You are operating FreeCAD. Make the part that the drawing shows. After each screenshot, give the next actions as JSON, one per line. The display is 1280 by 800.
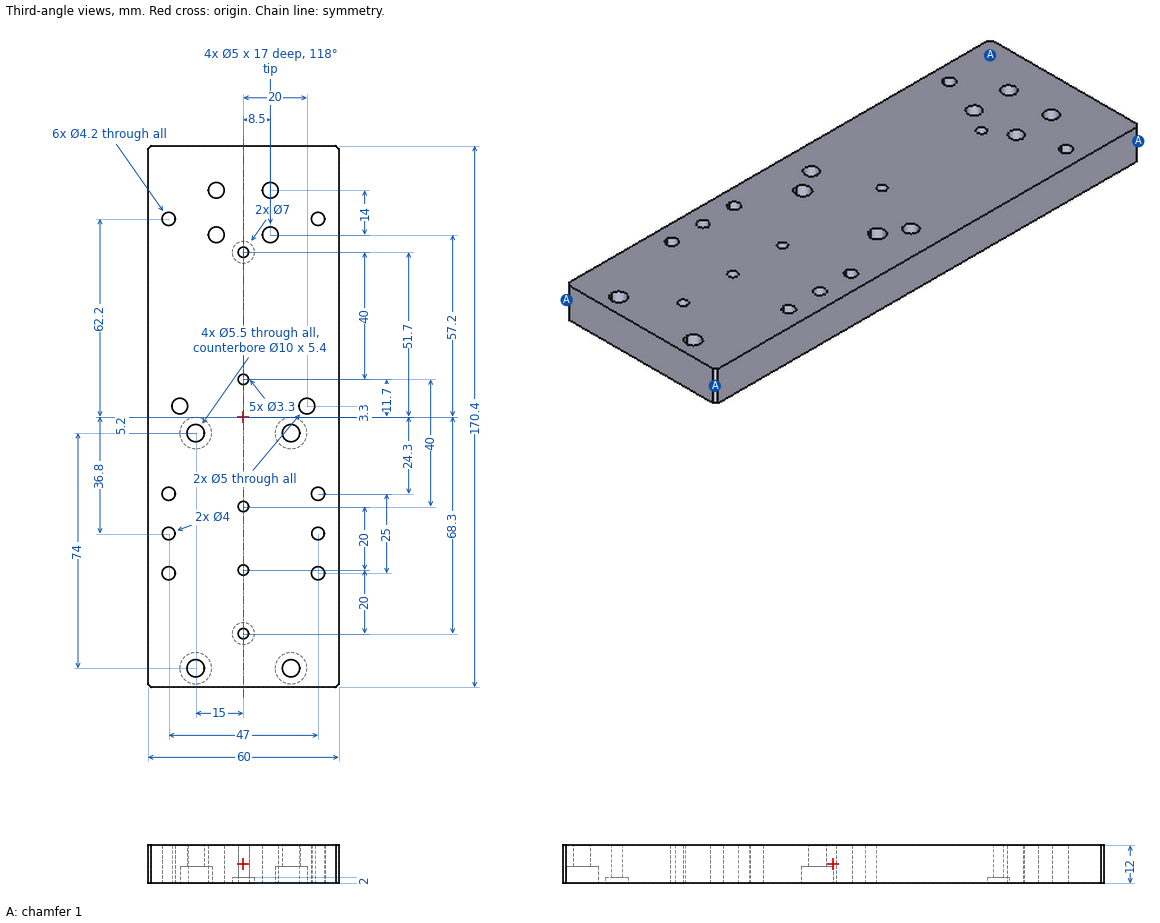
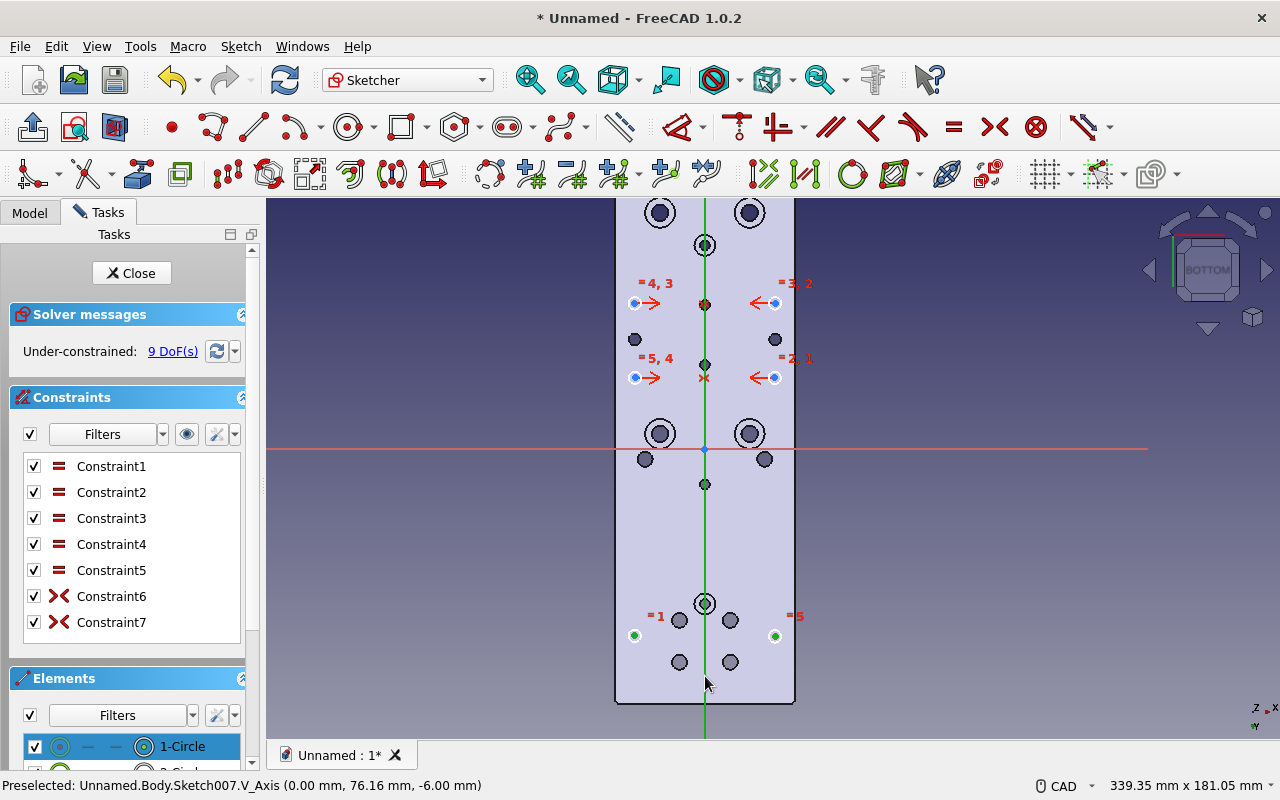
{"action": "left_click", "coordinate": [995, 128]}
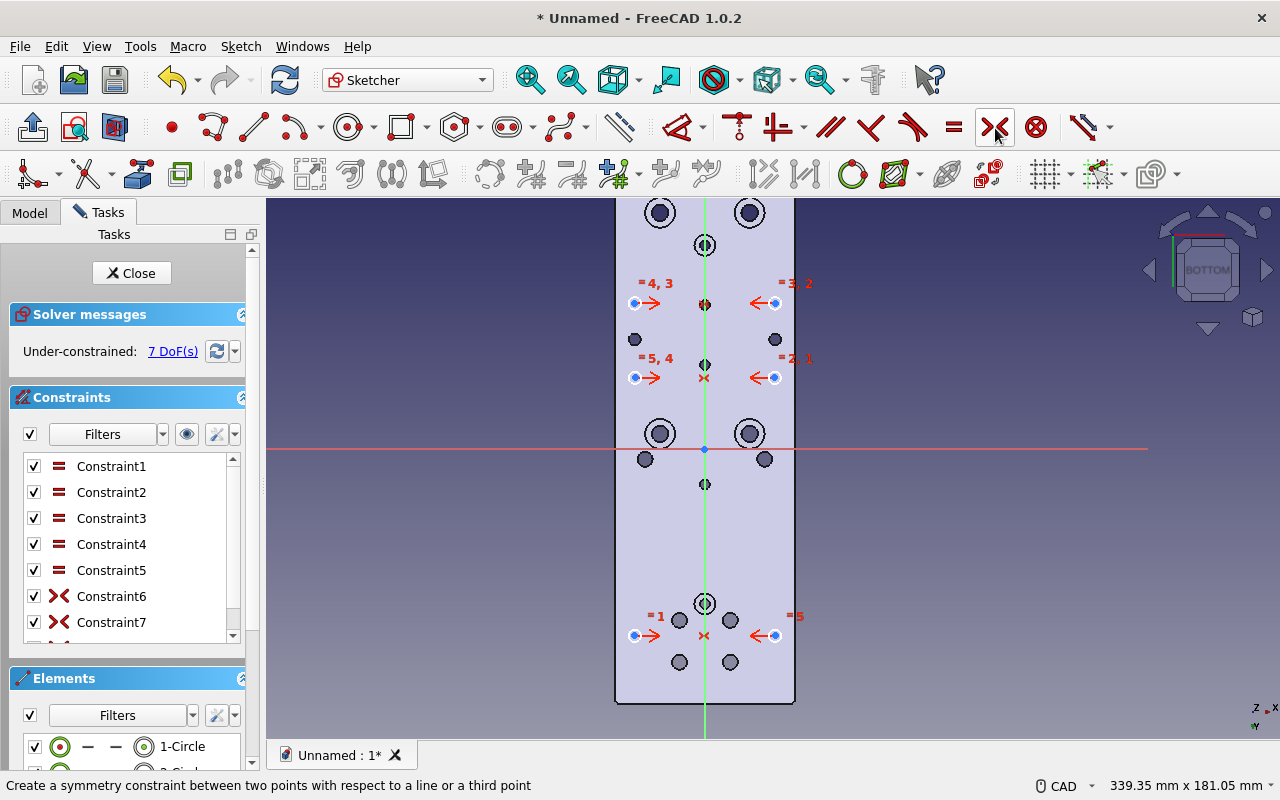
{"action": "left_click", "coordinate": [676, 128]}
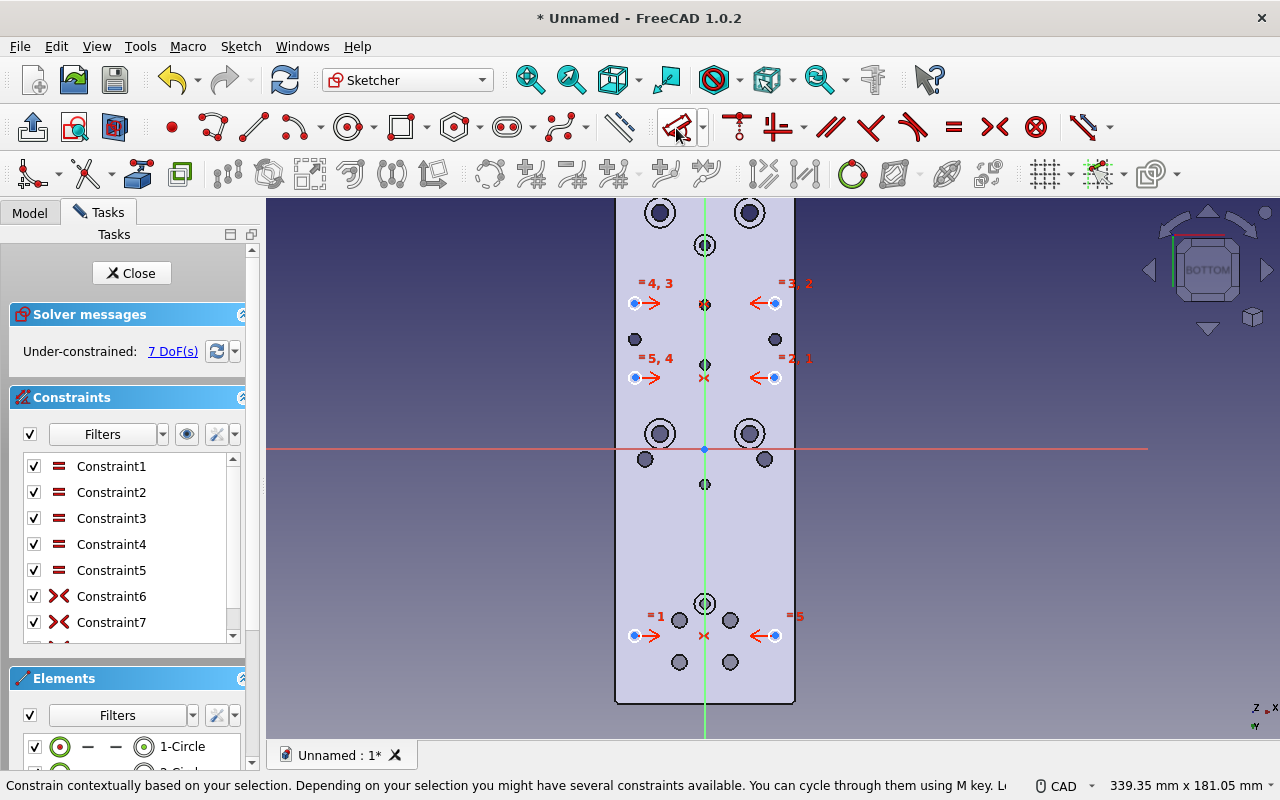
{"action": "scroll", "coordinate": [635, 642], "scroll_direction": "up", "scroll_amount": 6}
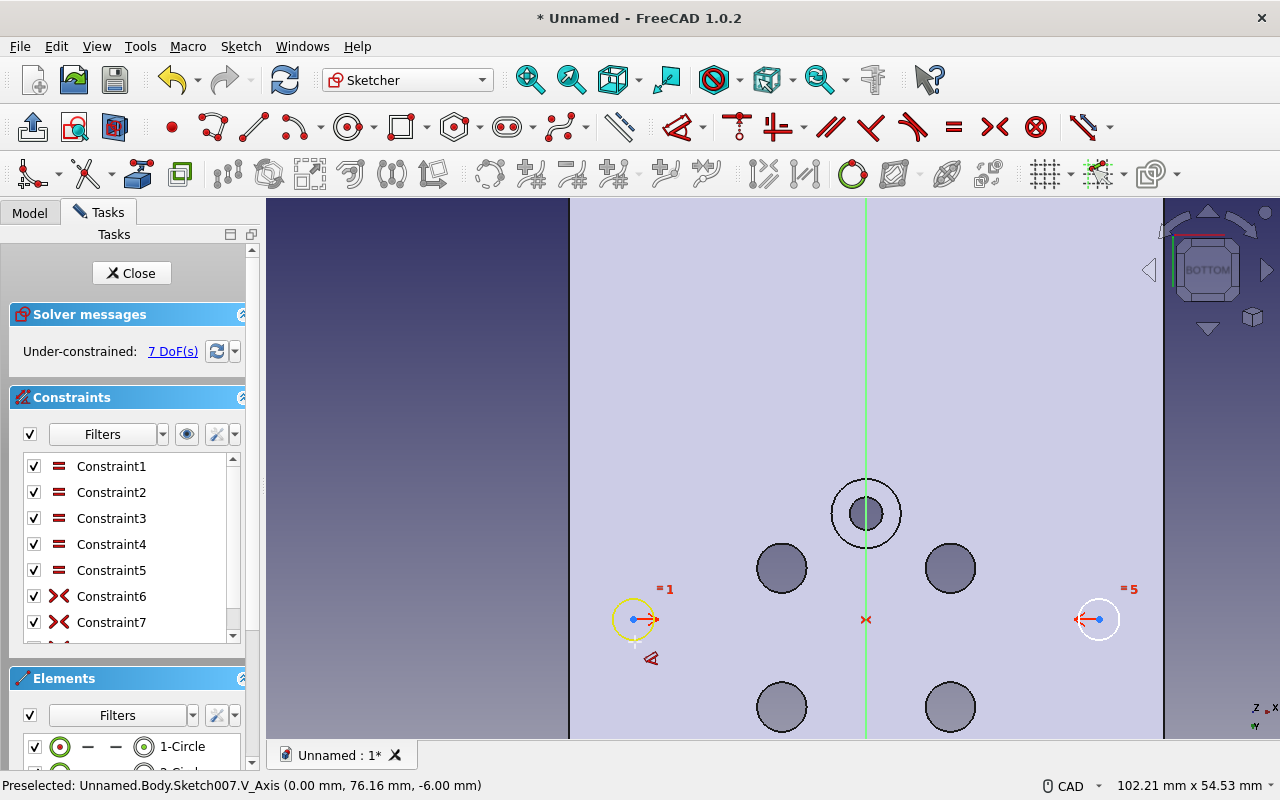
{"action": "left_click", "coordinate": [633, 640]}
{"action": "left_click", "coordinate": [632, 672]}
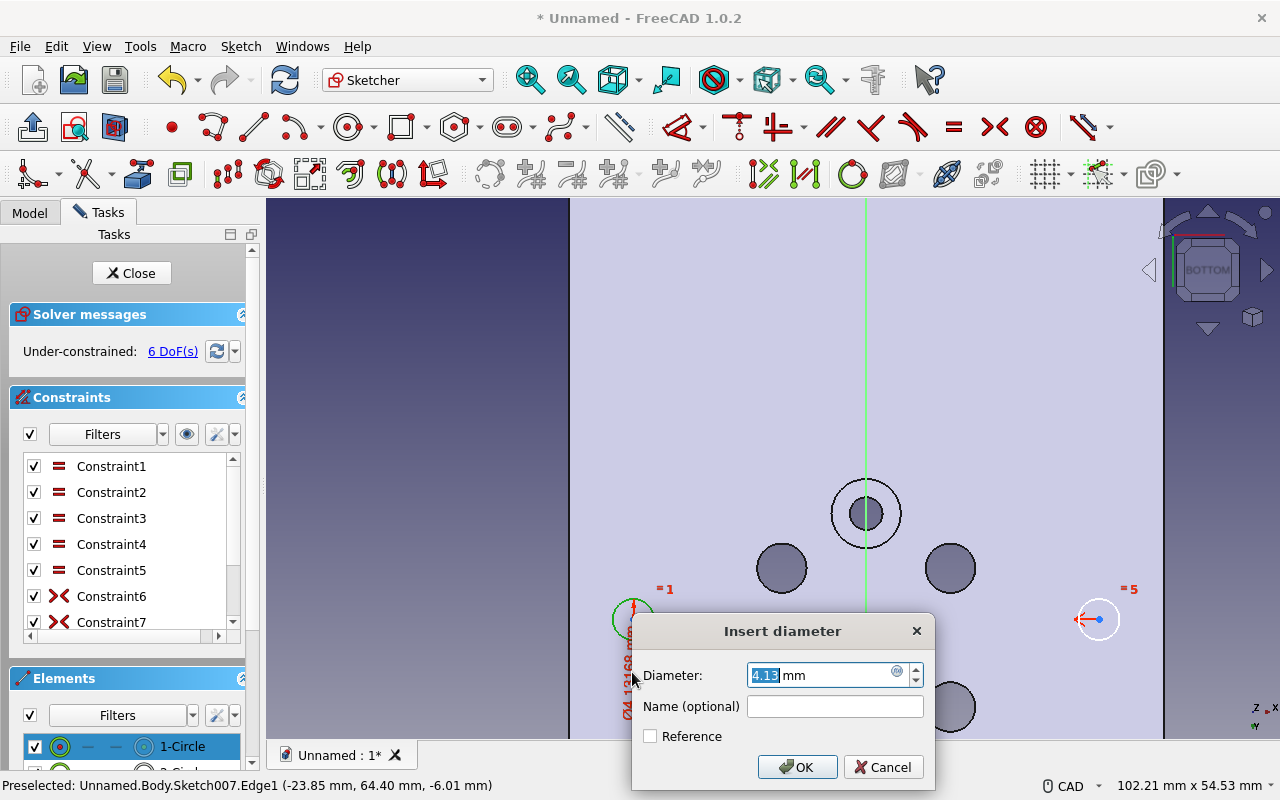
{"action": "type", "text": "4.2"}
{"action": "key", "text": "Return"}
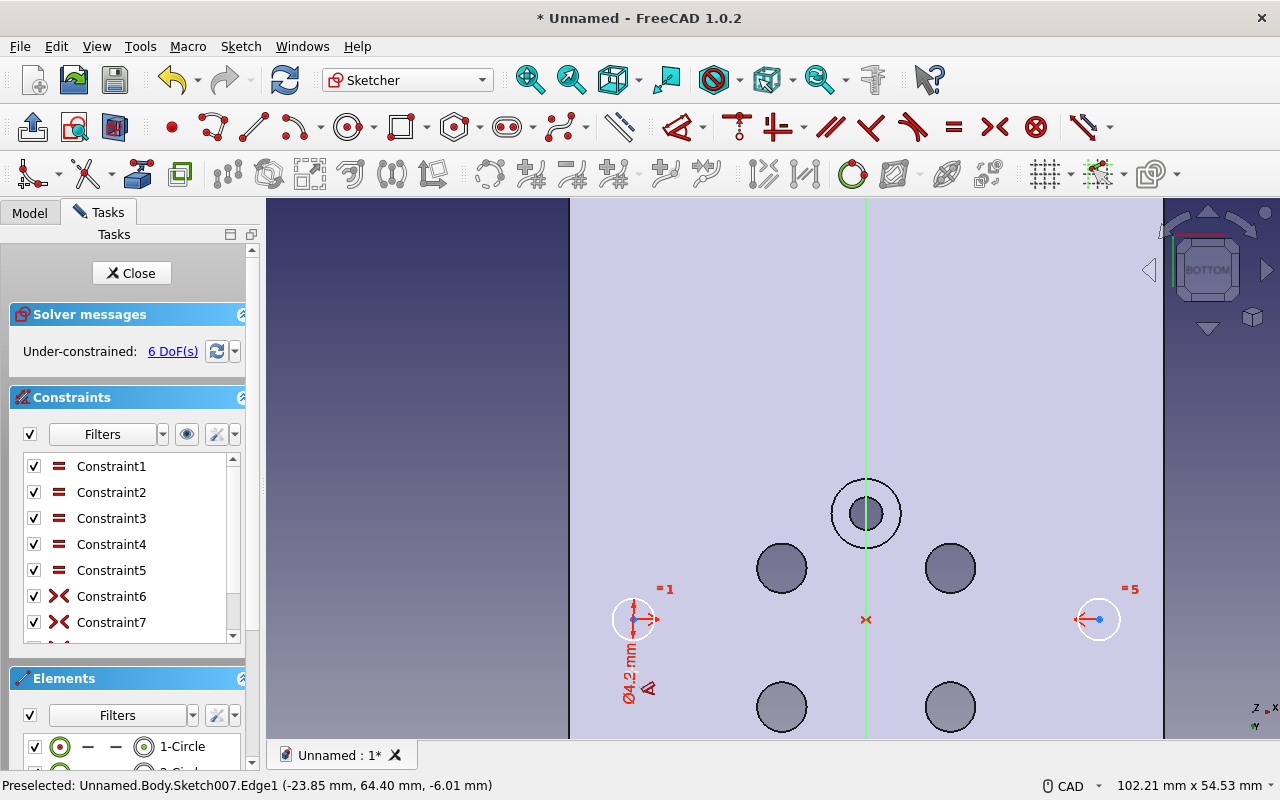
{"action": "left_click", "coordinate": [633, 619]}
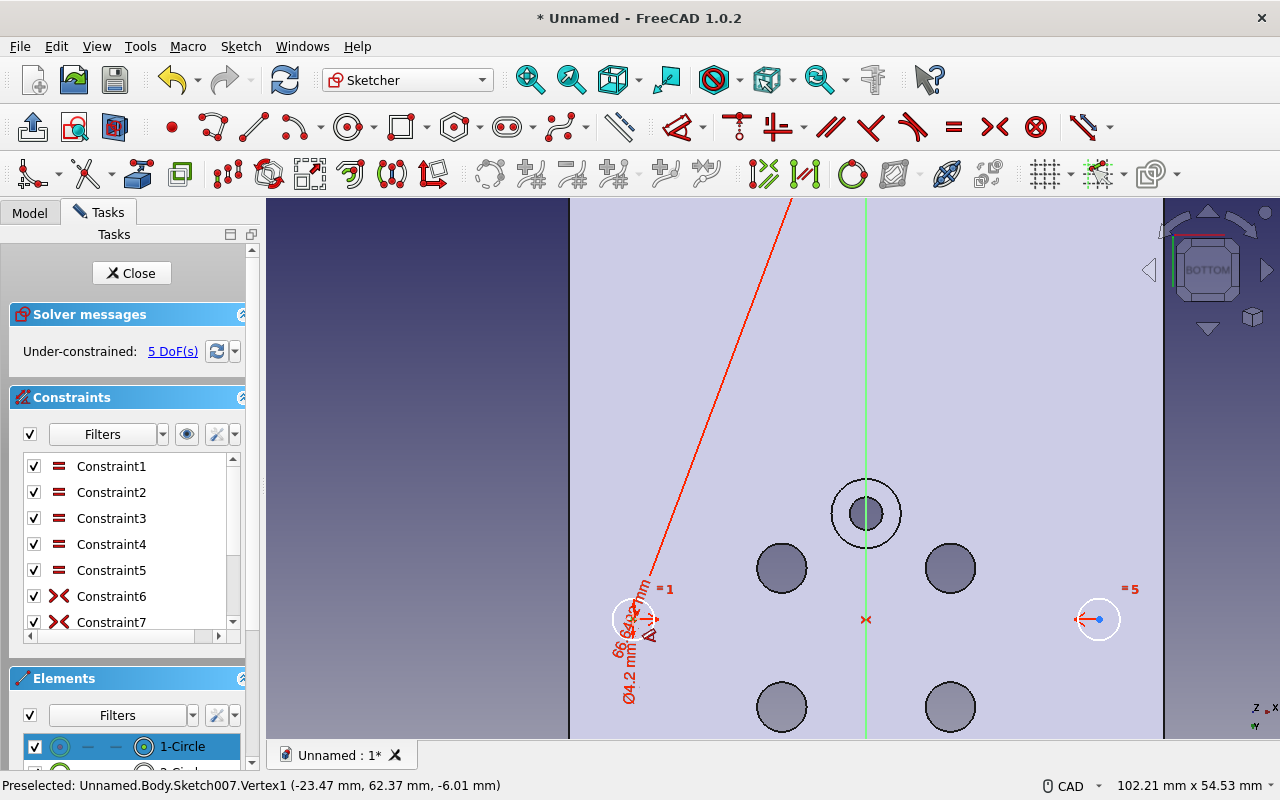
{"action": "scroll", "coordinate": [635, 643], "scroll_direction": "down", "scroll_amount": 6}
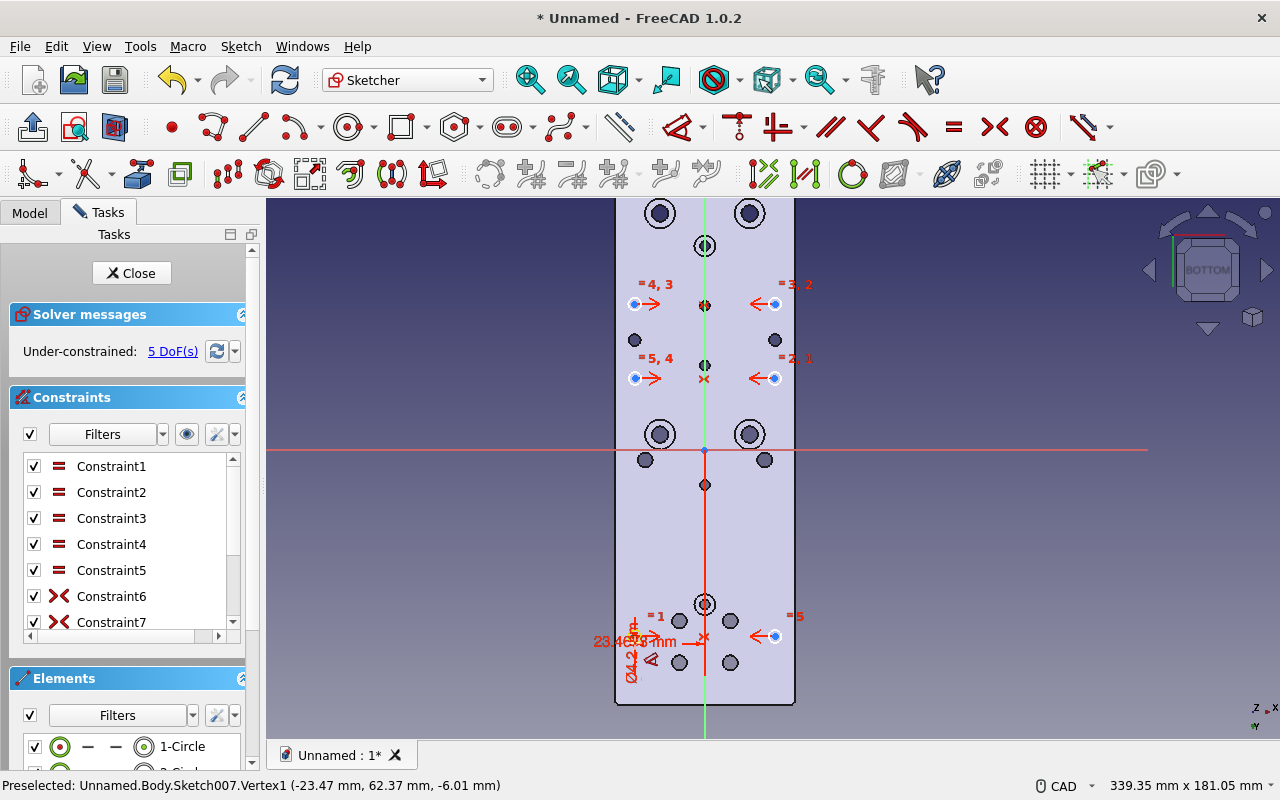
{"action": "left_click", "coordinate": [775, 378]}
{"action": "left_click", "coordinate": [737, 670]}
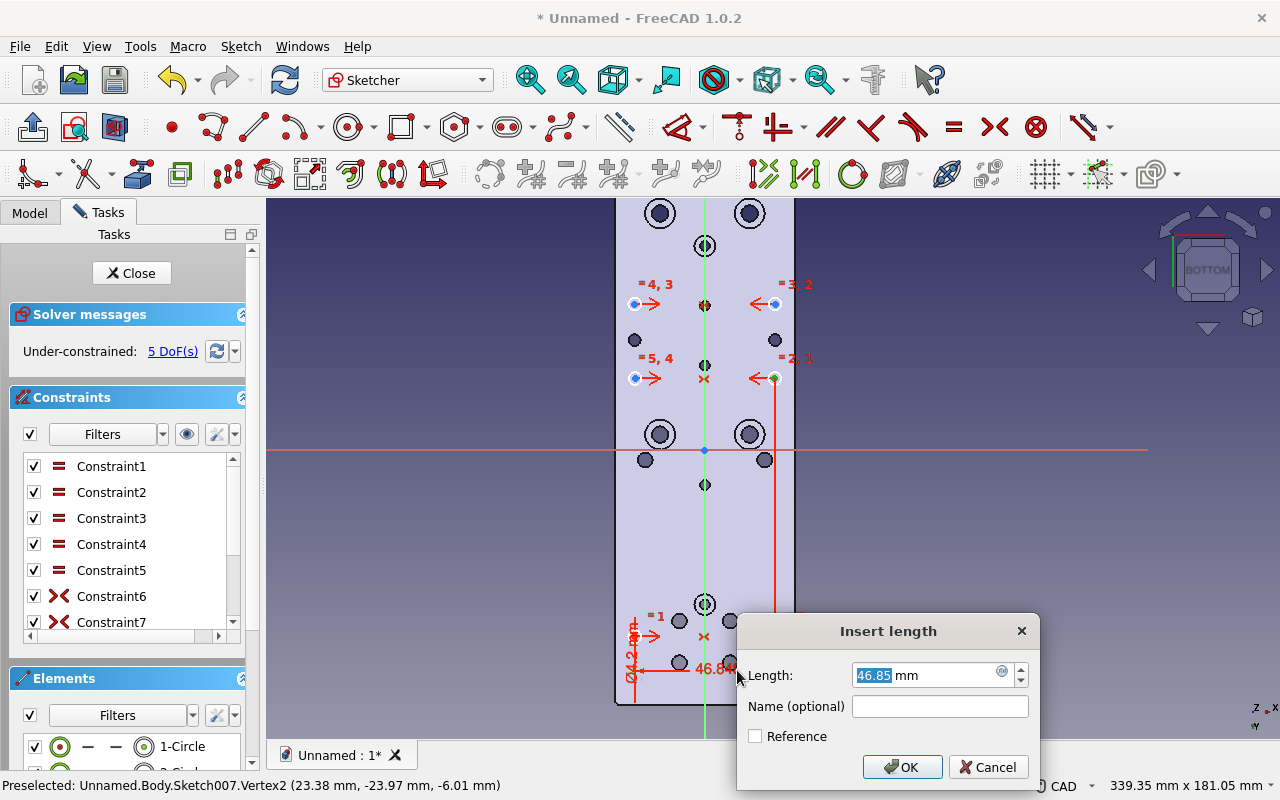
{"action": "type", "text": "47"}
{"action": "key", "text": "Return"}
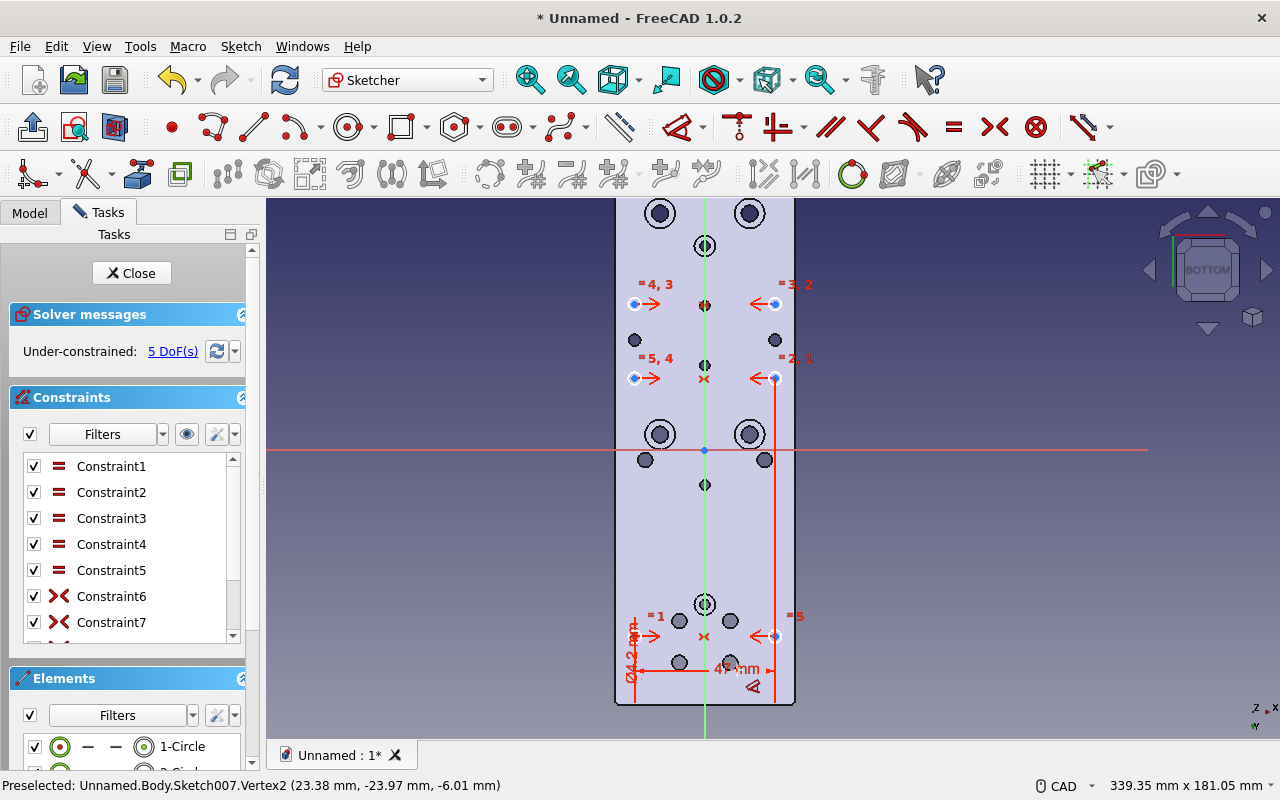
{"action": "left_click", "coordinate": [635, 636]}